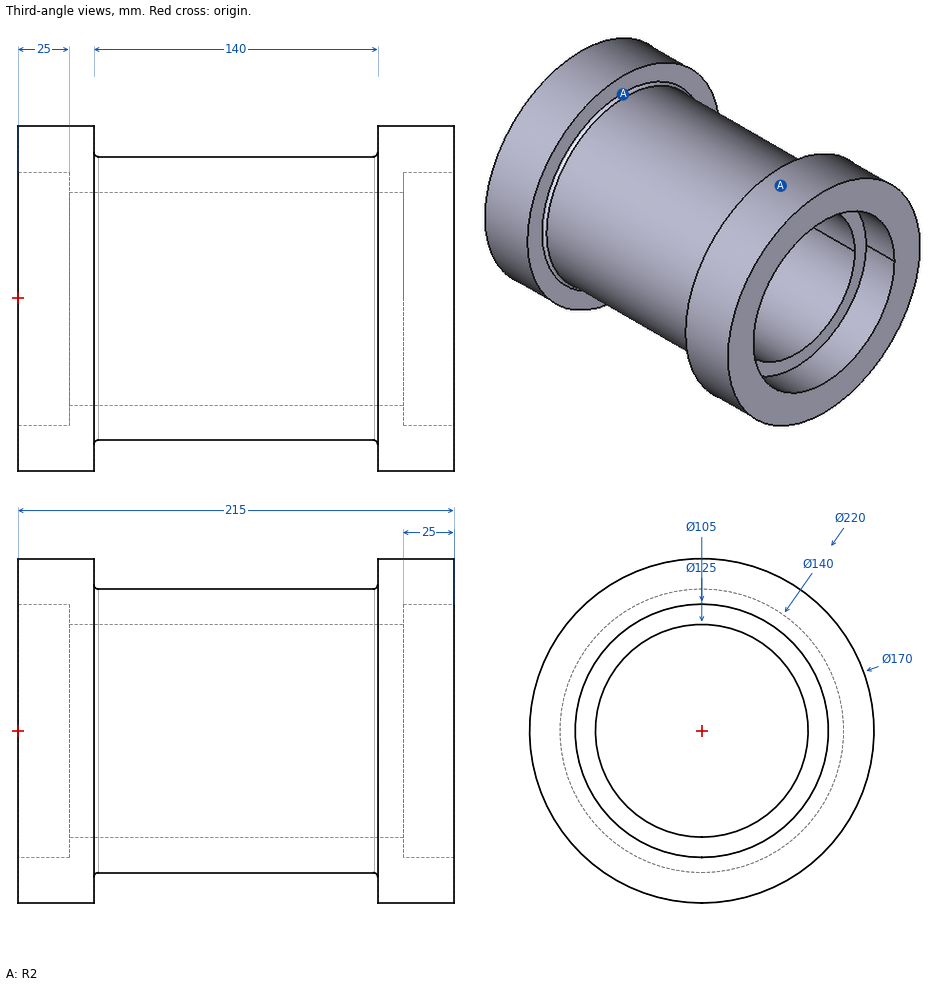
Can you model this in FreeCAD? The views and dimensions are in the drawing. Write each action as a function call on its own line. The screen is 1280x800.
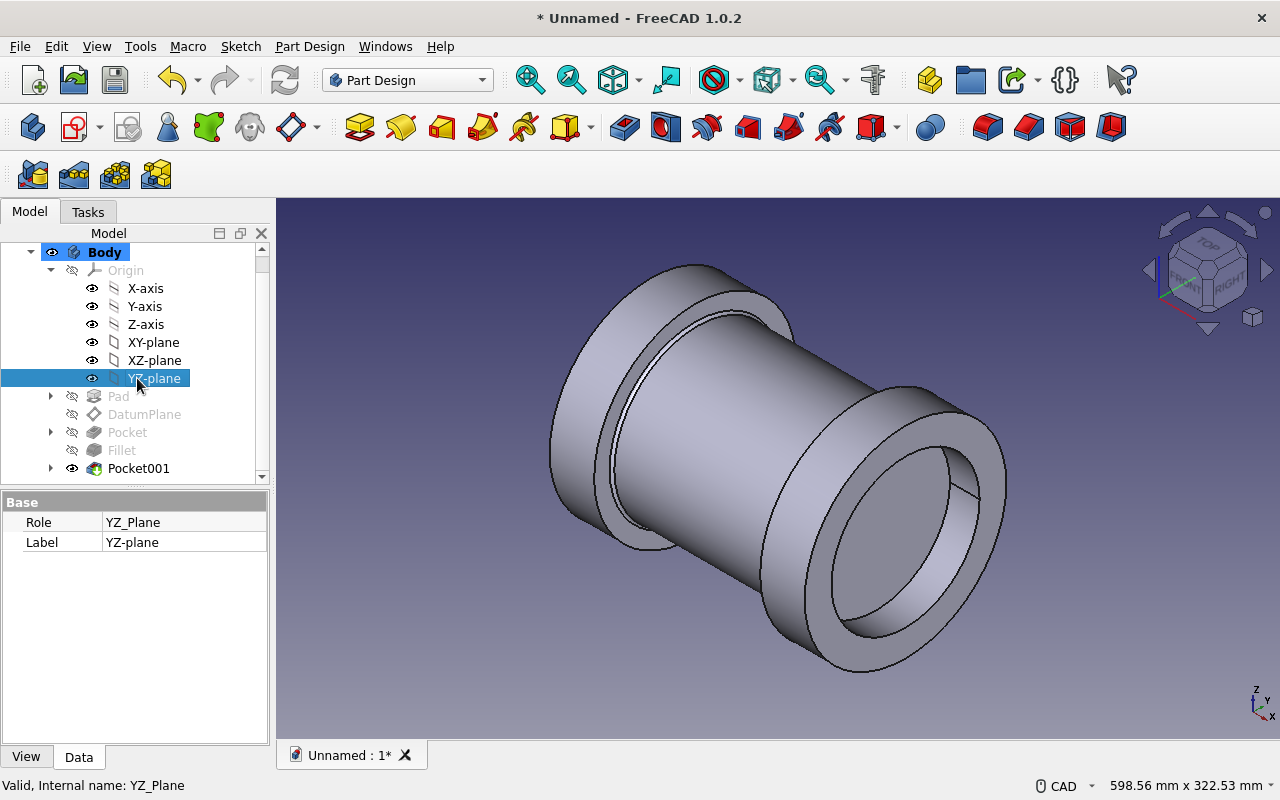
click(290, 128)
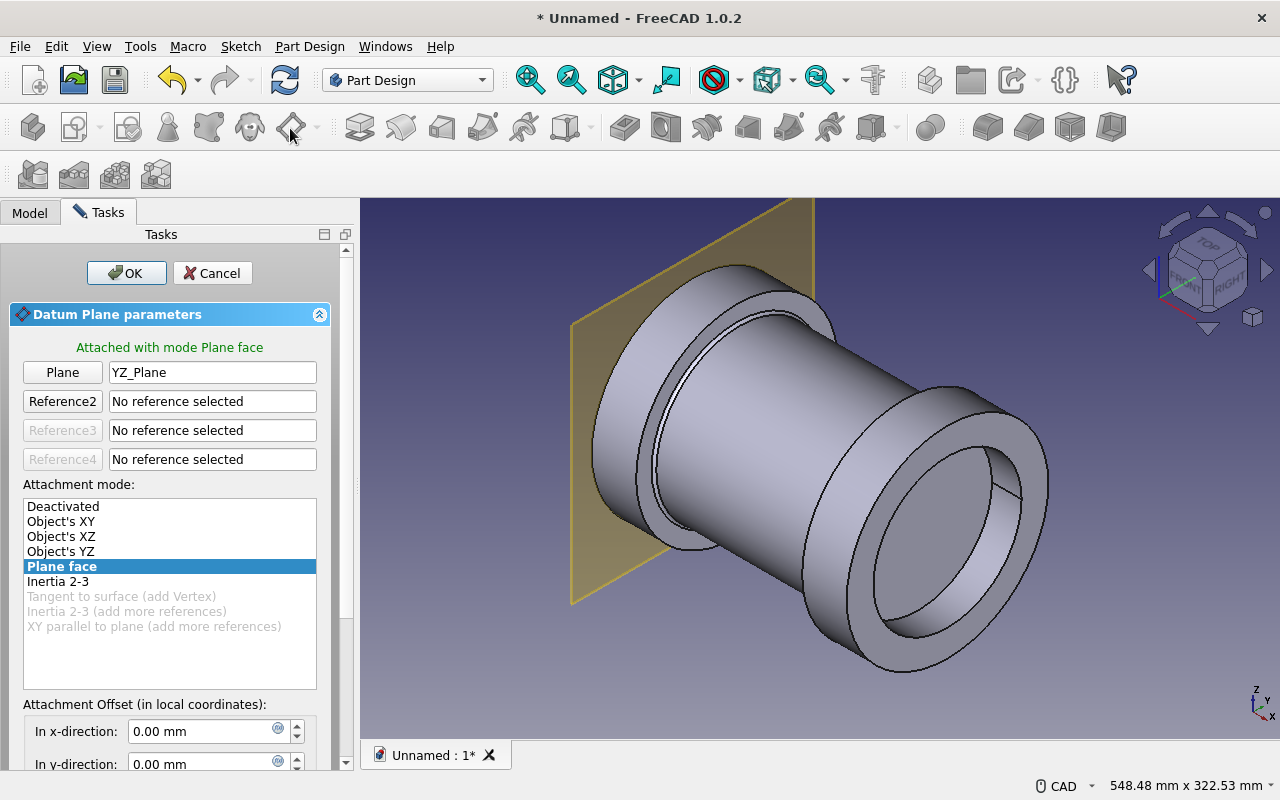
scroll(346, 507, down, 2)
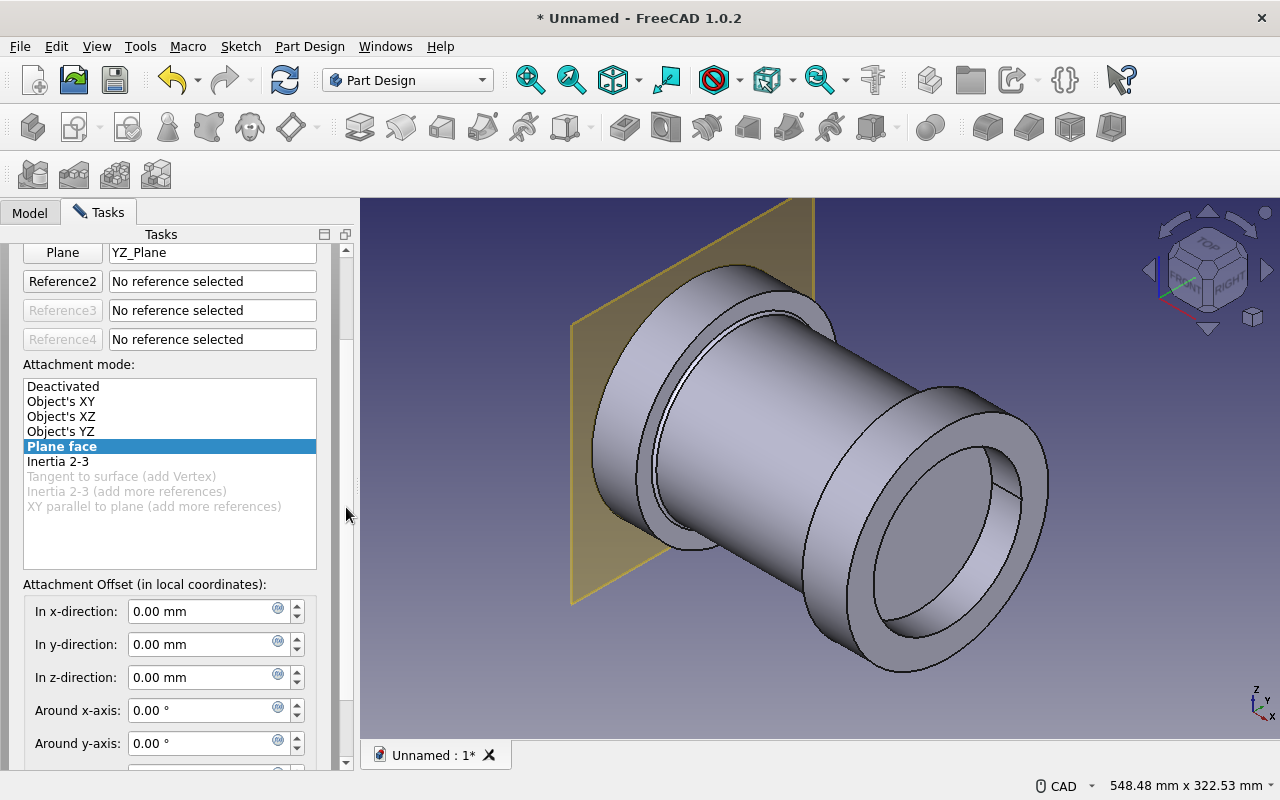
triple_click(210, 678)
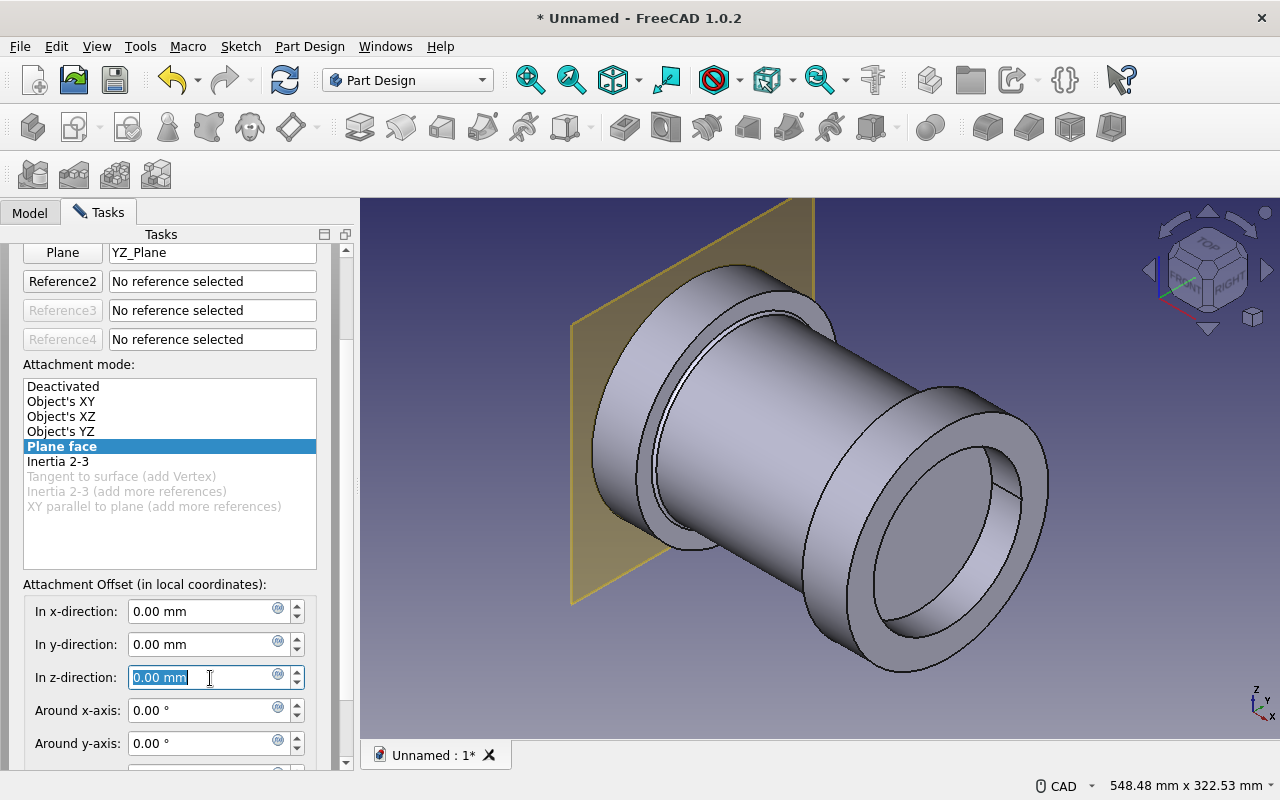
text(25)
key(Tab)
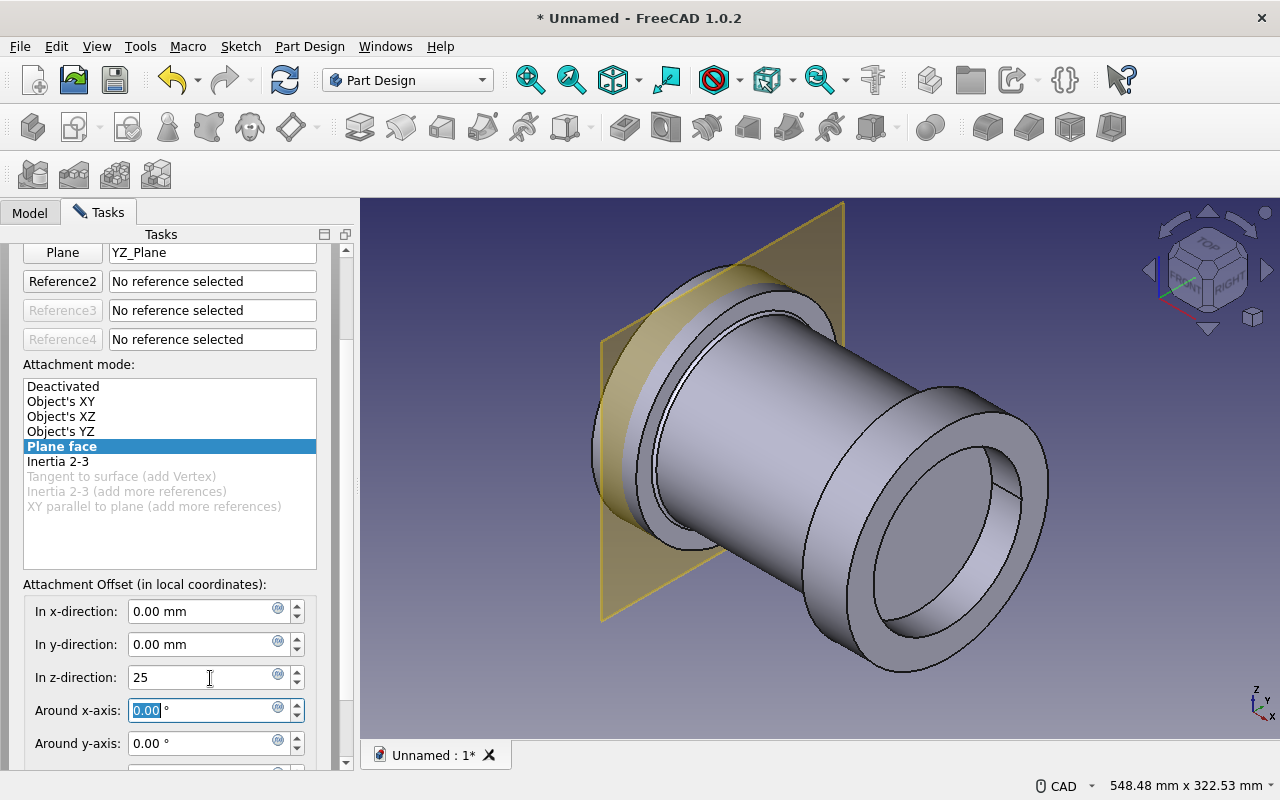
scroll(346, 507, up, 3)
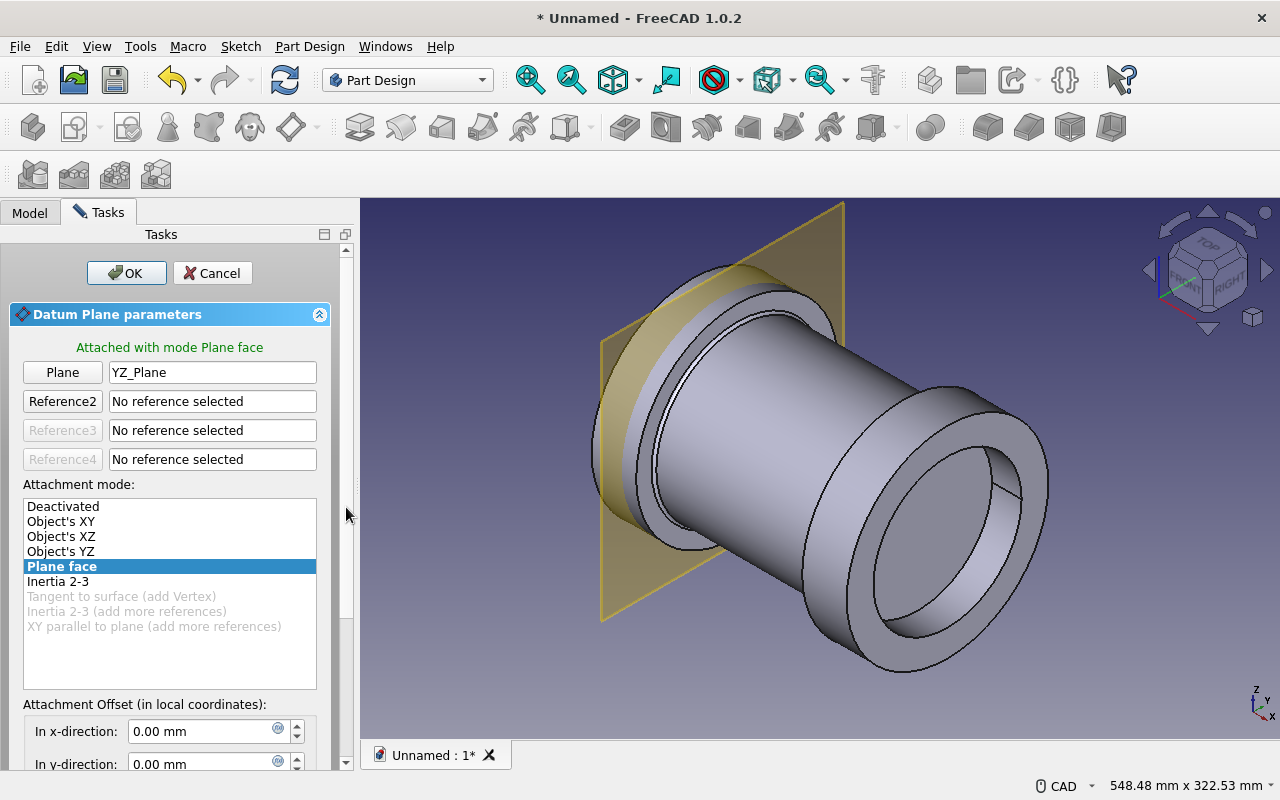
click(127, 273)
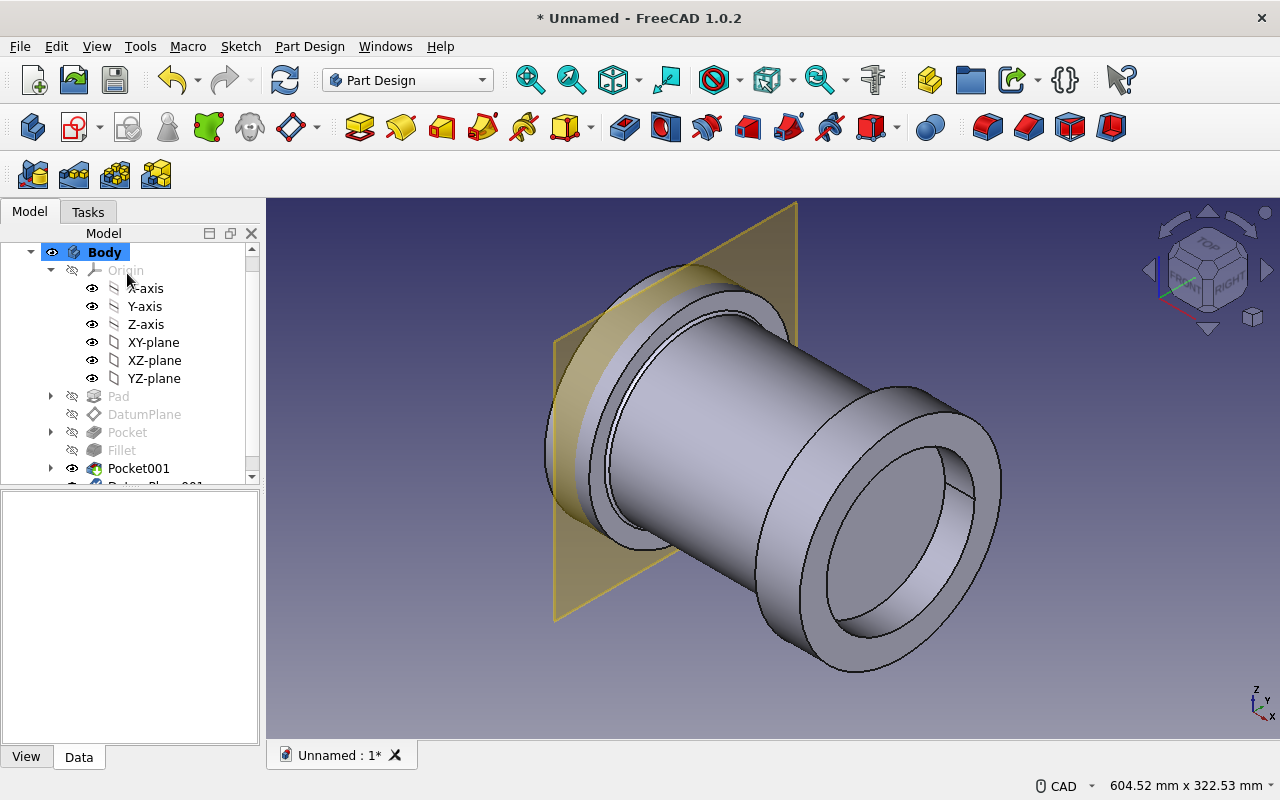
scroll(121, 356, down, 3)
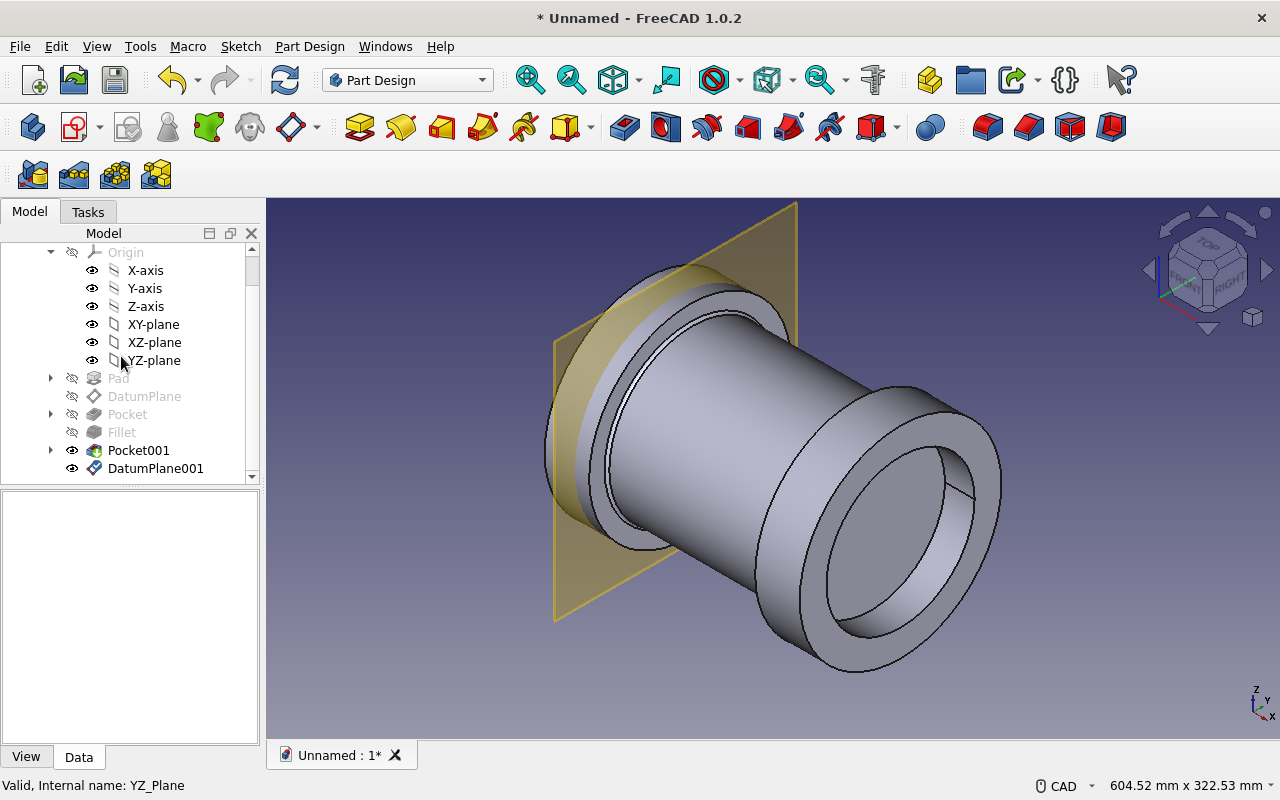
click(117, 468)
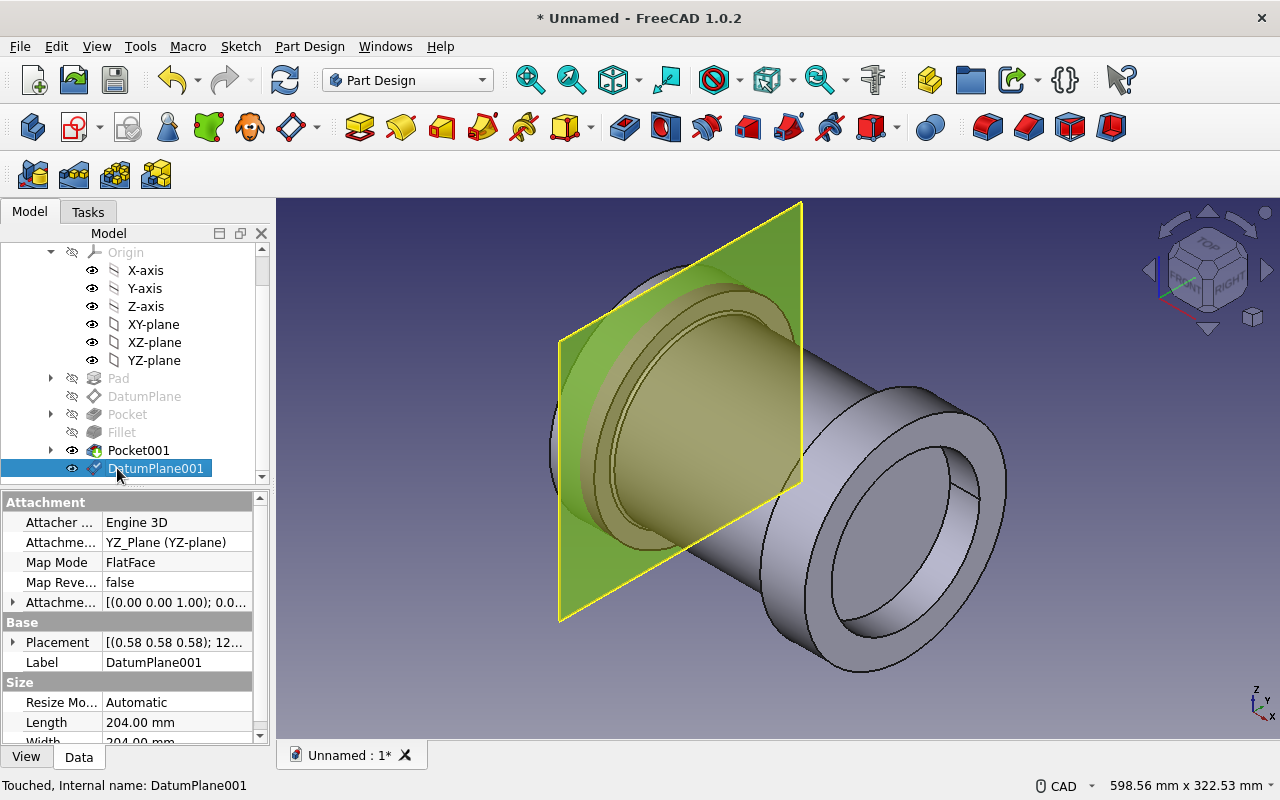
click(74, 128)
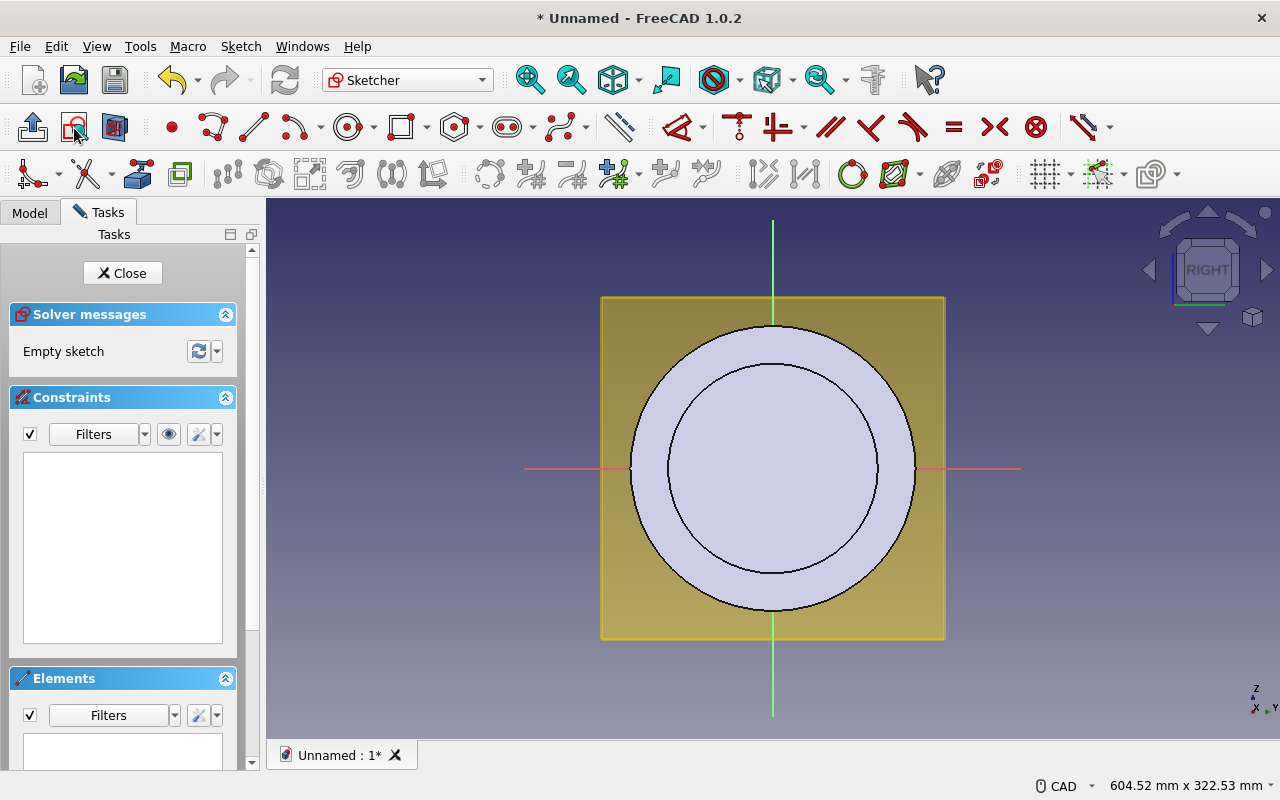
click(115, 128)